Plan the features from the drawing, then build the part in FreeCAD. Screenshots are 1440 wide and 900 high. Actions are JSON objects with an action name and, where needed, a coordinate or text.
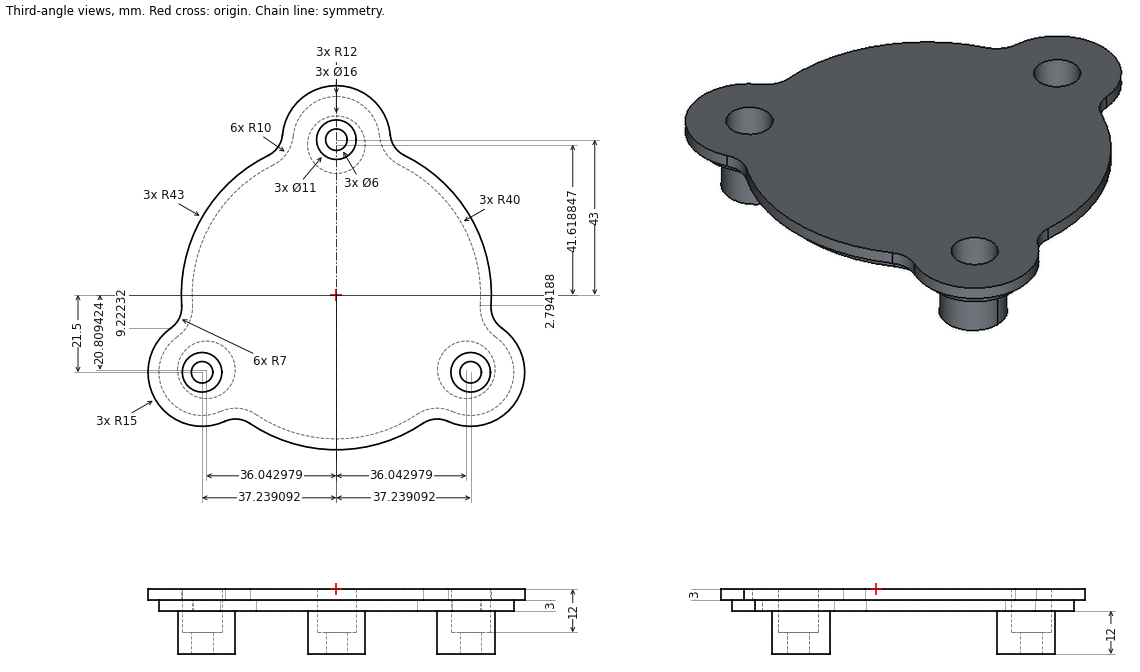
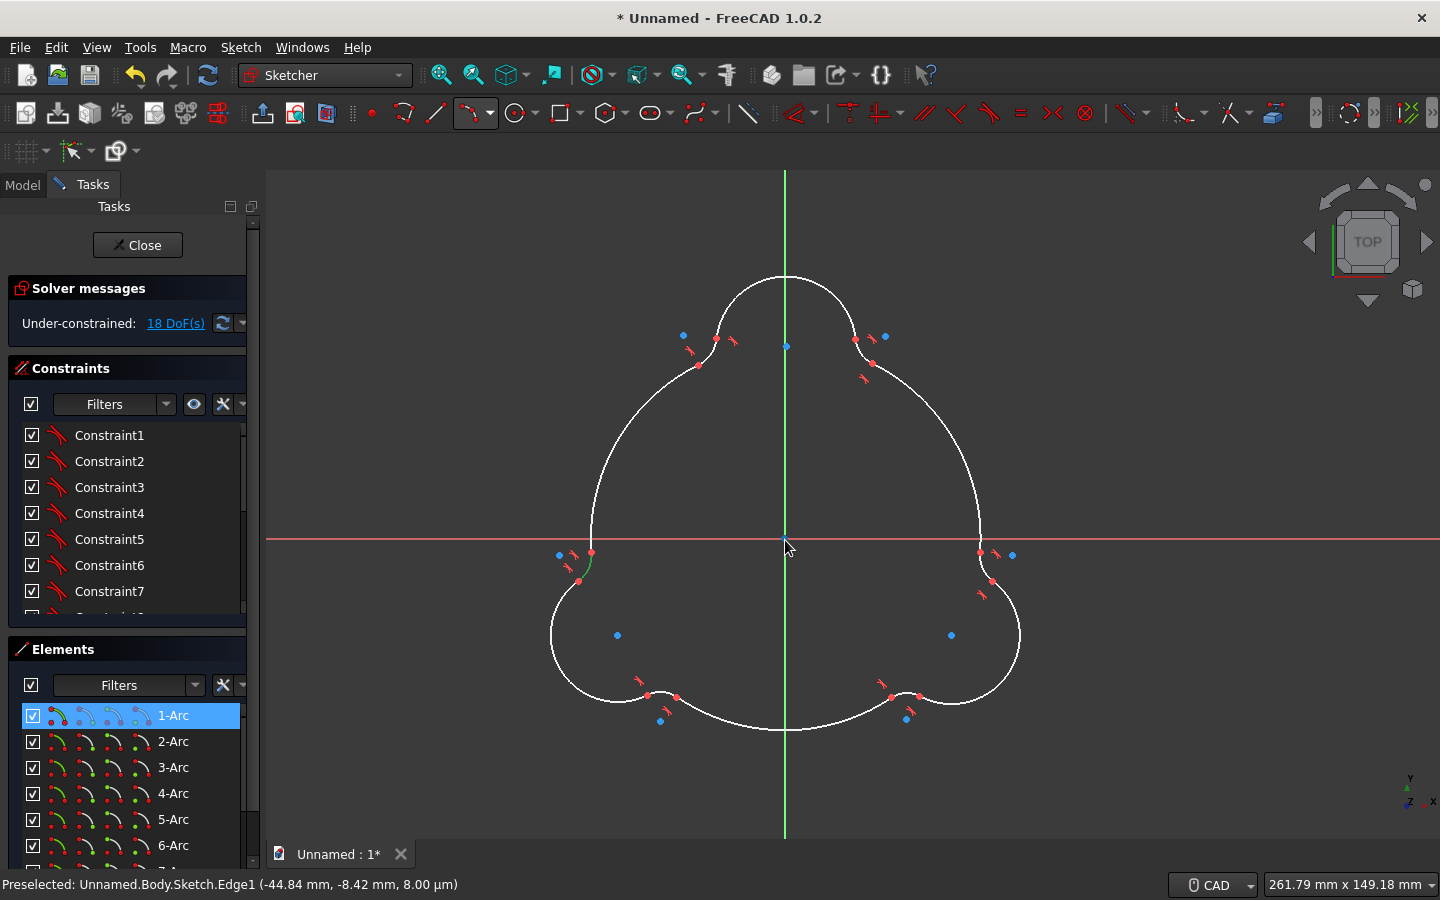
{"action": "scroll", "coordinate": [669, 693], "scroll_direction": "up", "scroll_amount": 2}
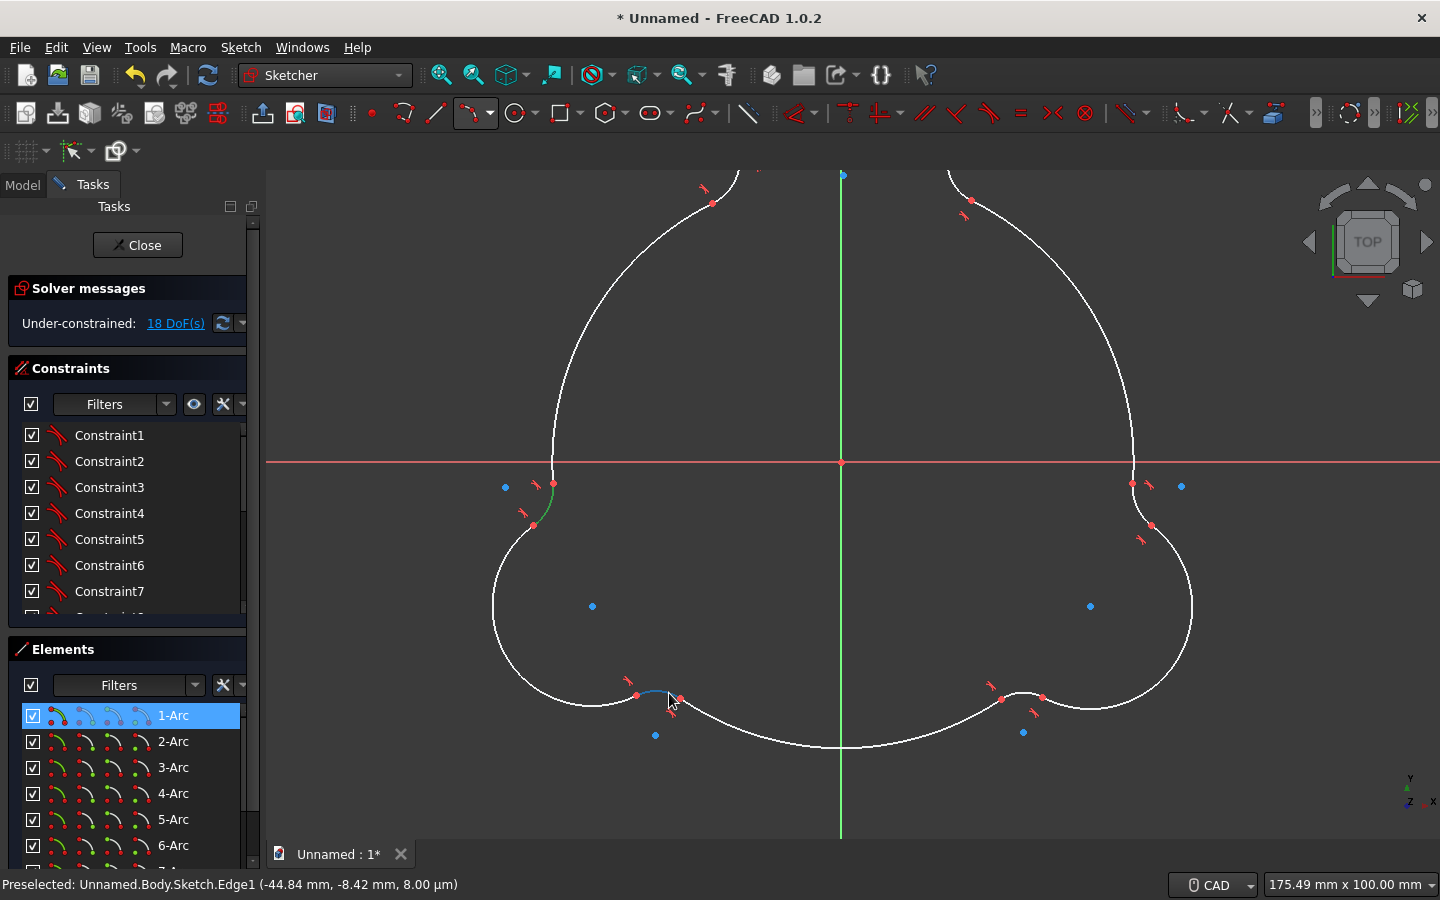
{"action": "left_click", "coordinate": [668, 693]}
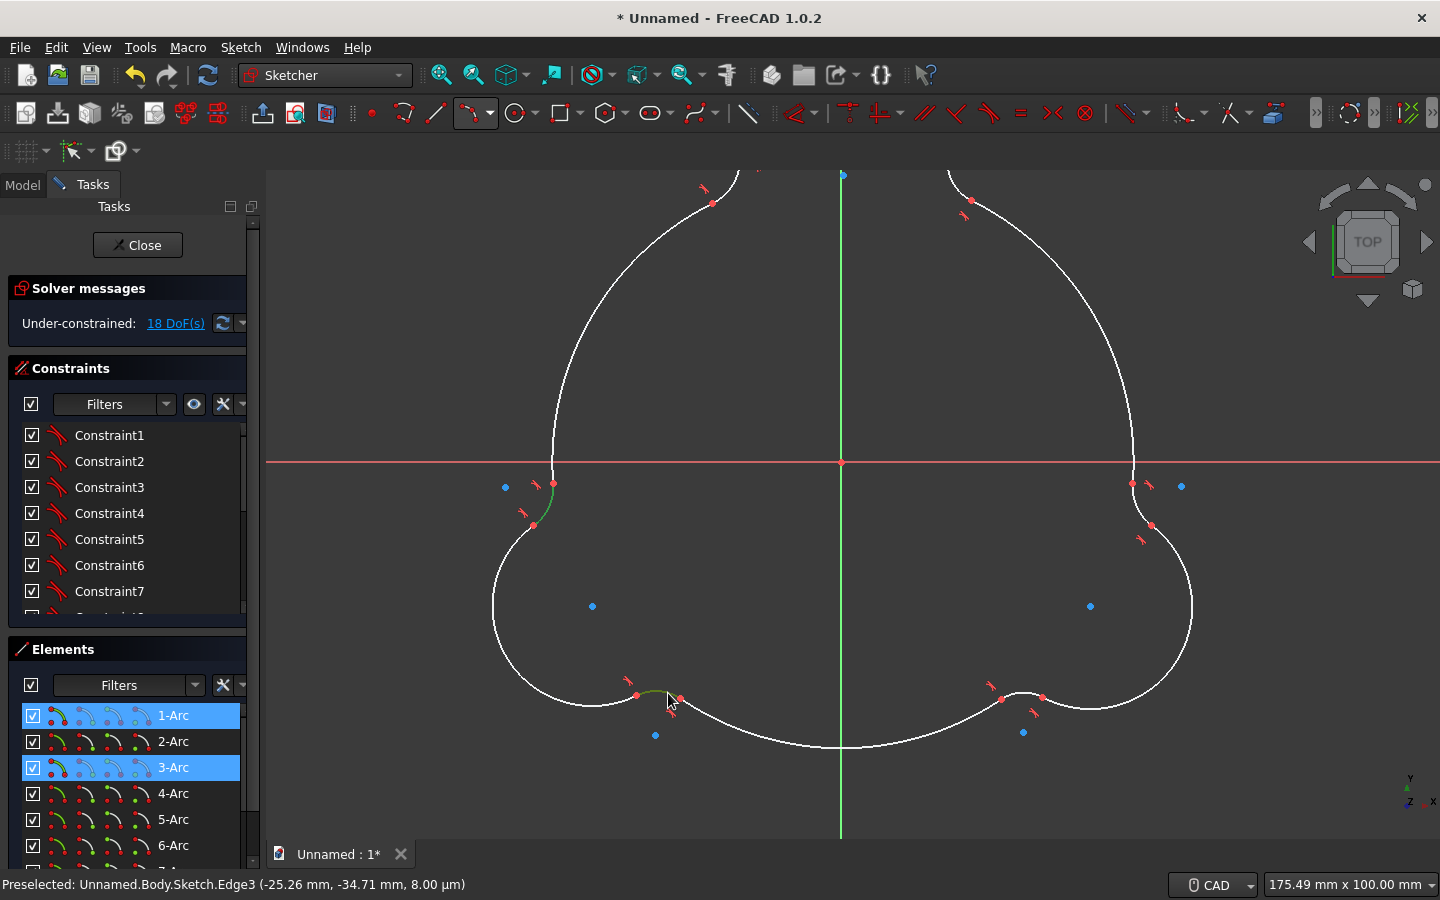
{"action": "left_click", "coordinate": [1030, 693]}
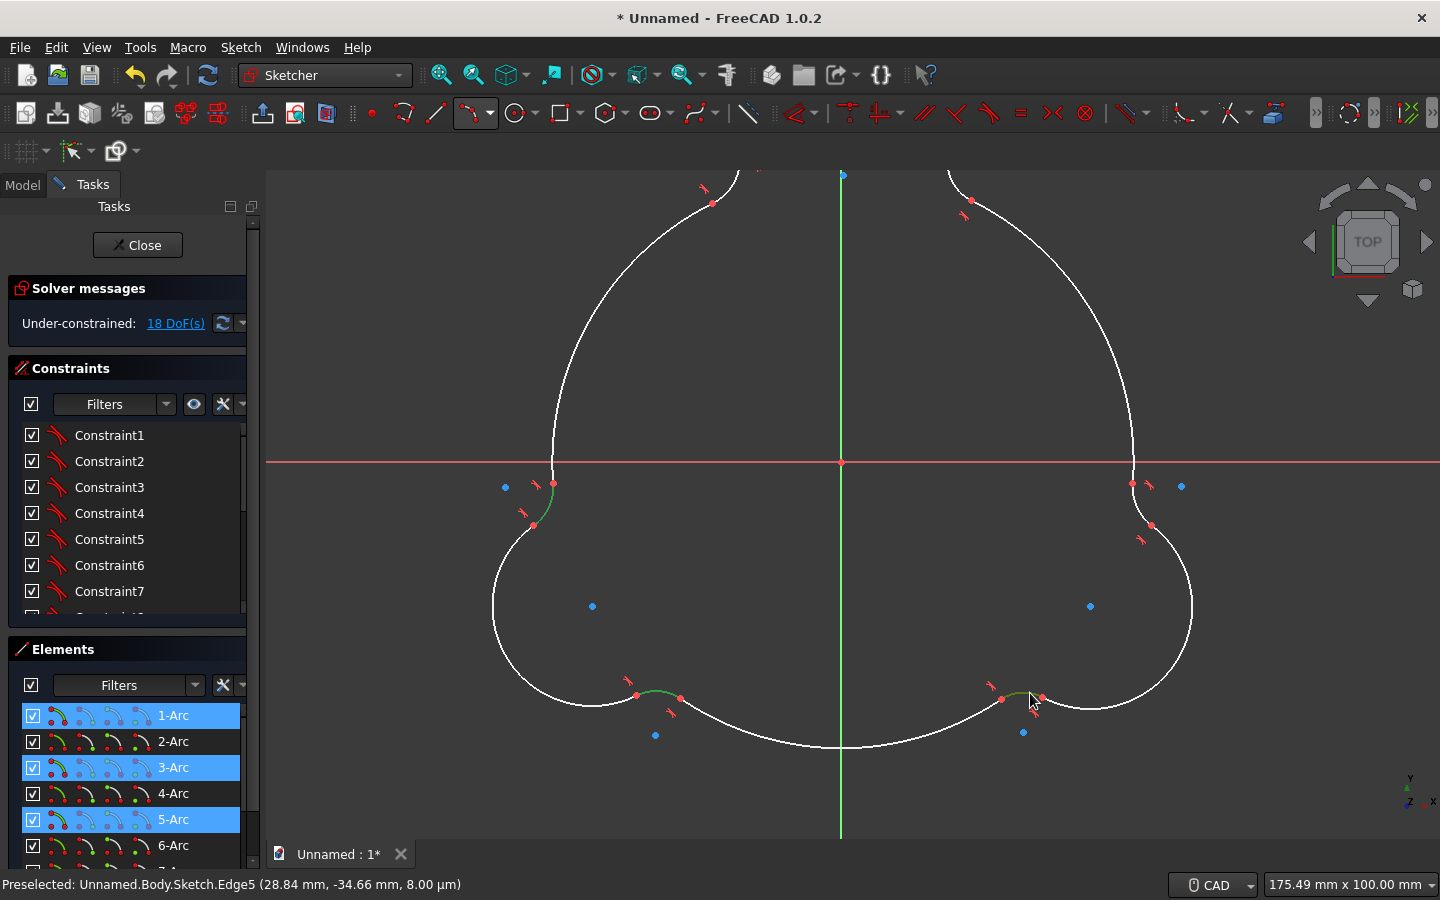
{"action": "left_click", "coordinate": [1134, 498]}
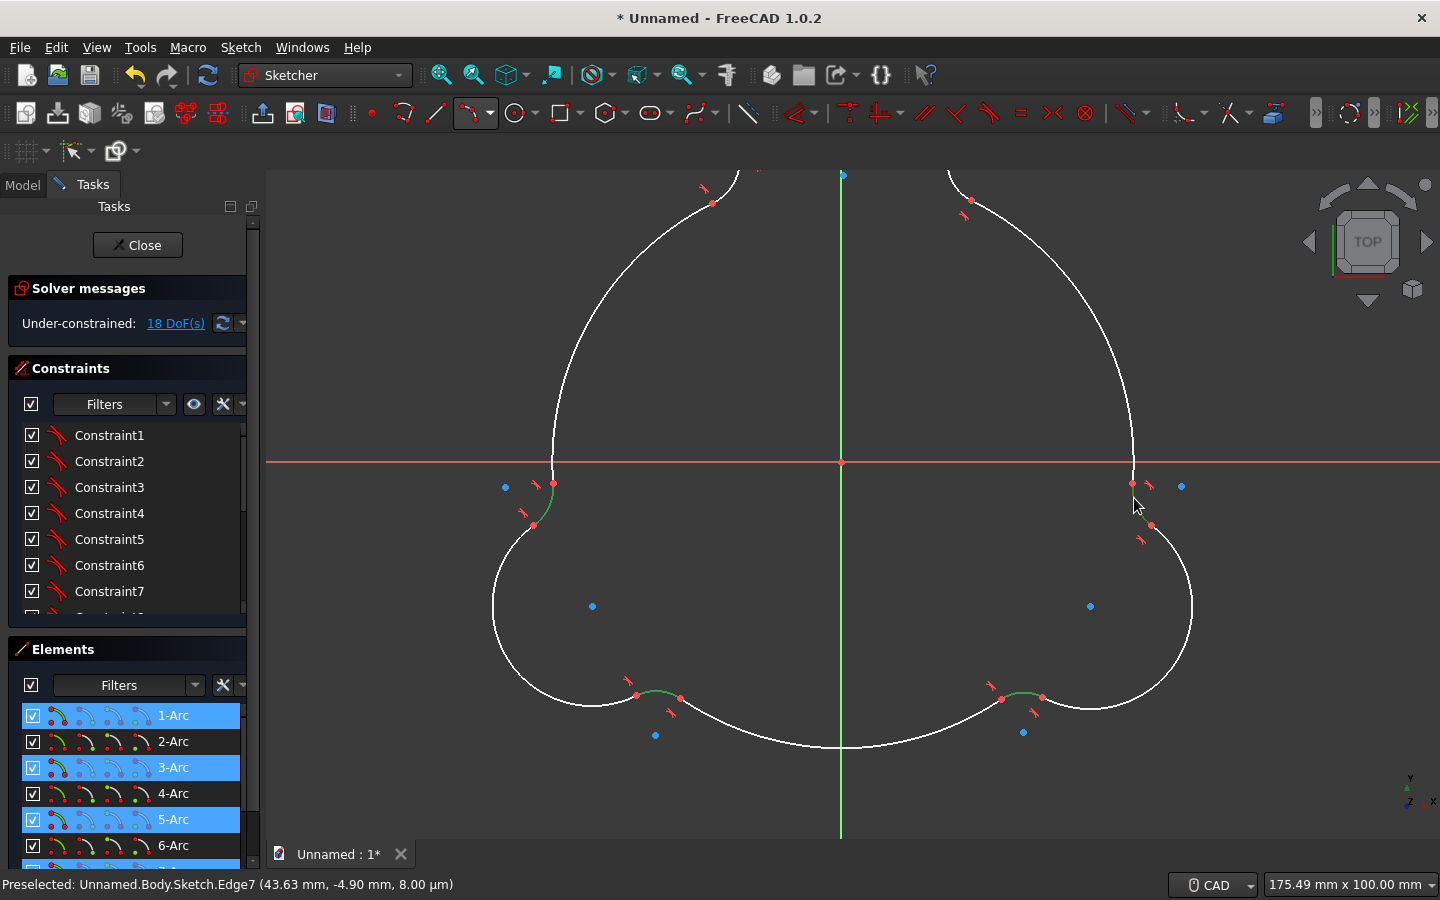
{"action": "scroll", "coordinate": [669, 693], "scroll_direction": "down", "scroll_amount": 2}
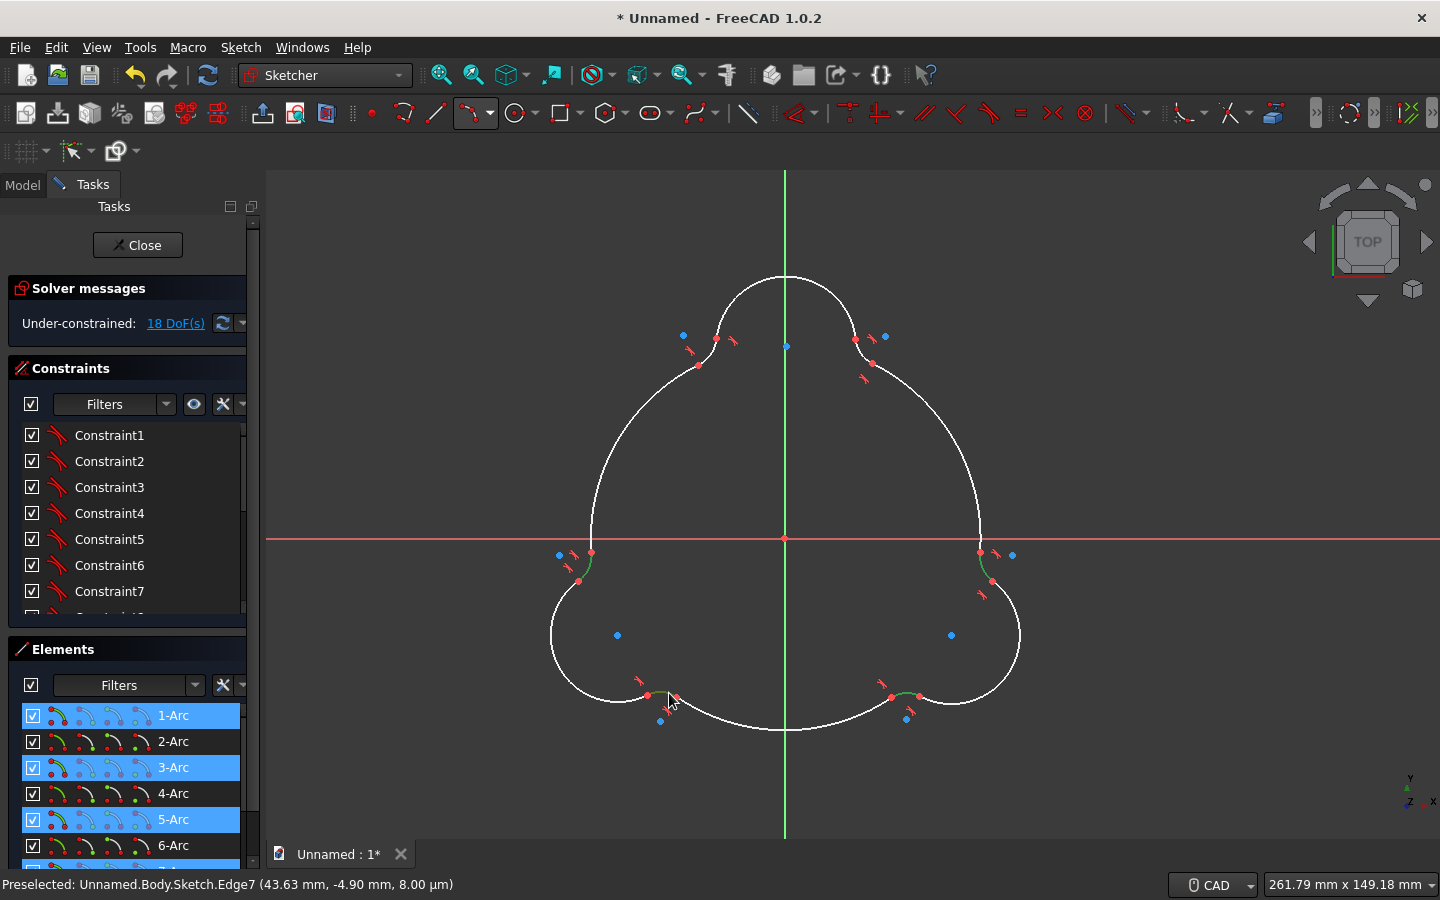
{"action": "scroll", "coordinate": [858, 348], "scroll_direction": "up", "scroll_amount": 3}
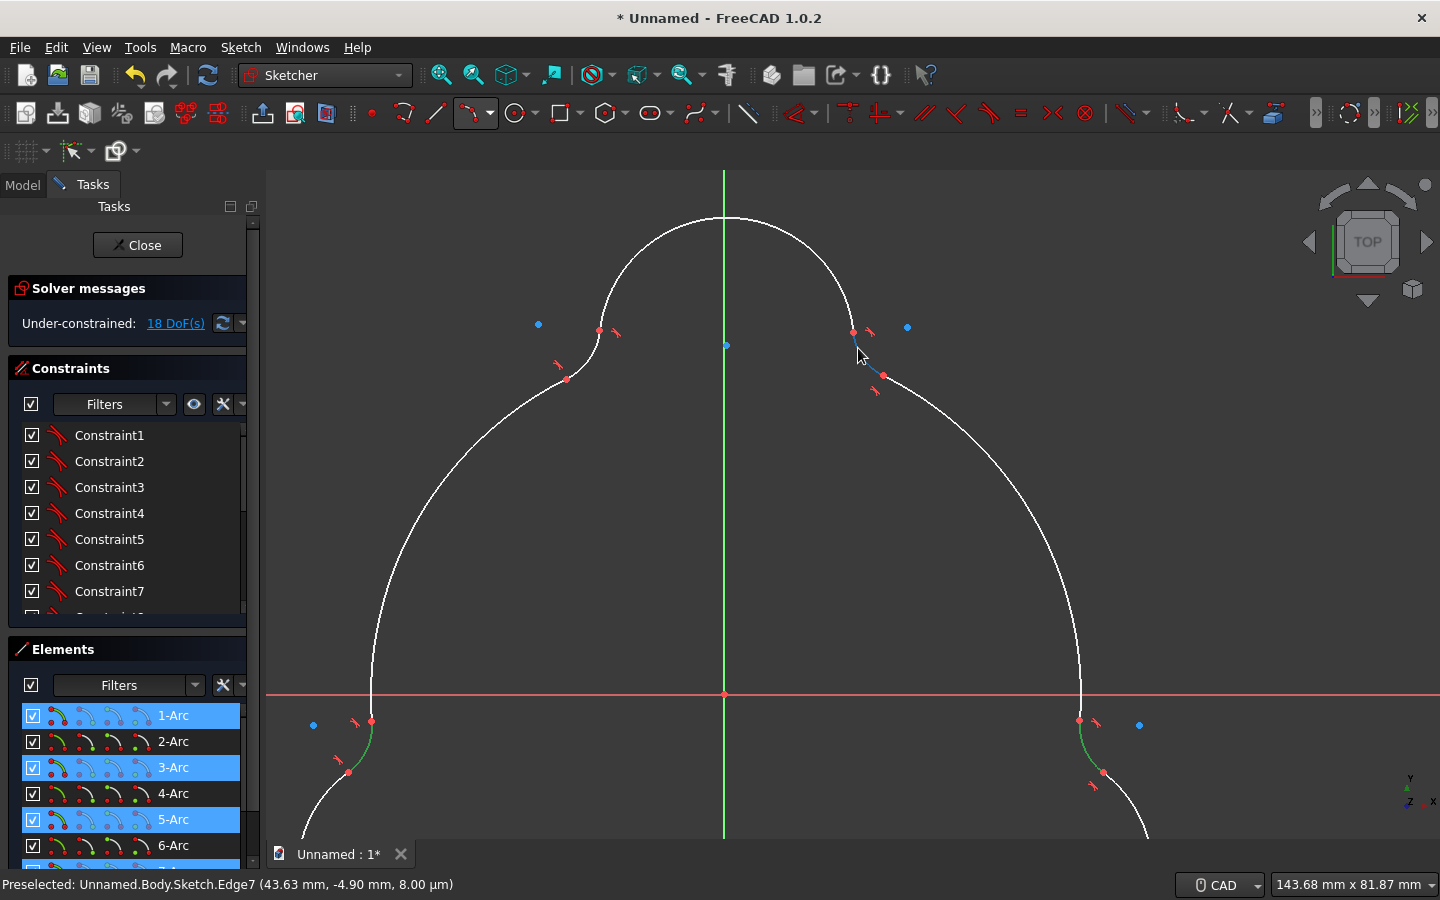
{"action": "left_click", "coordinate": [858, 348]}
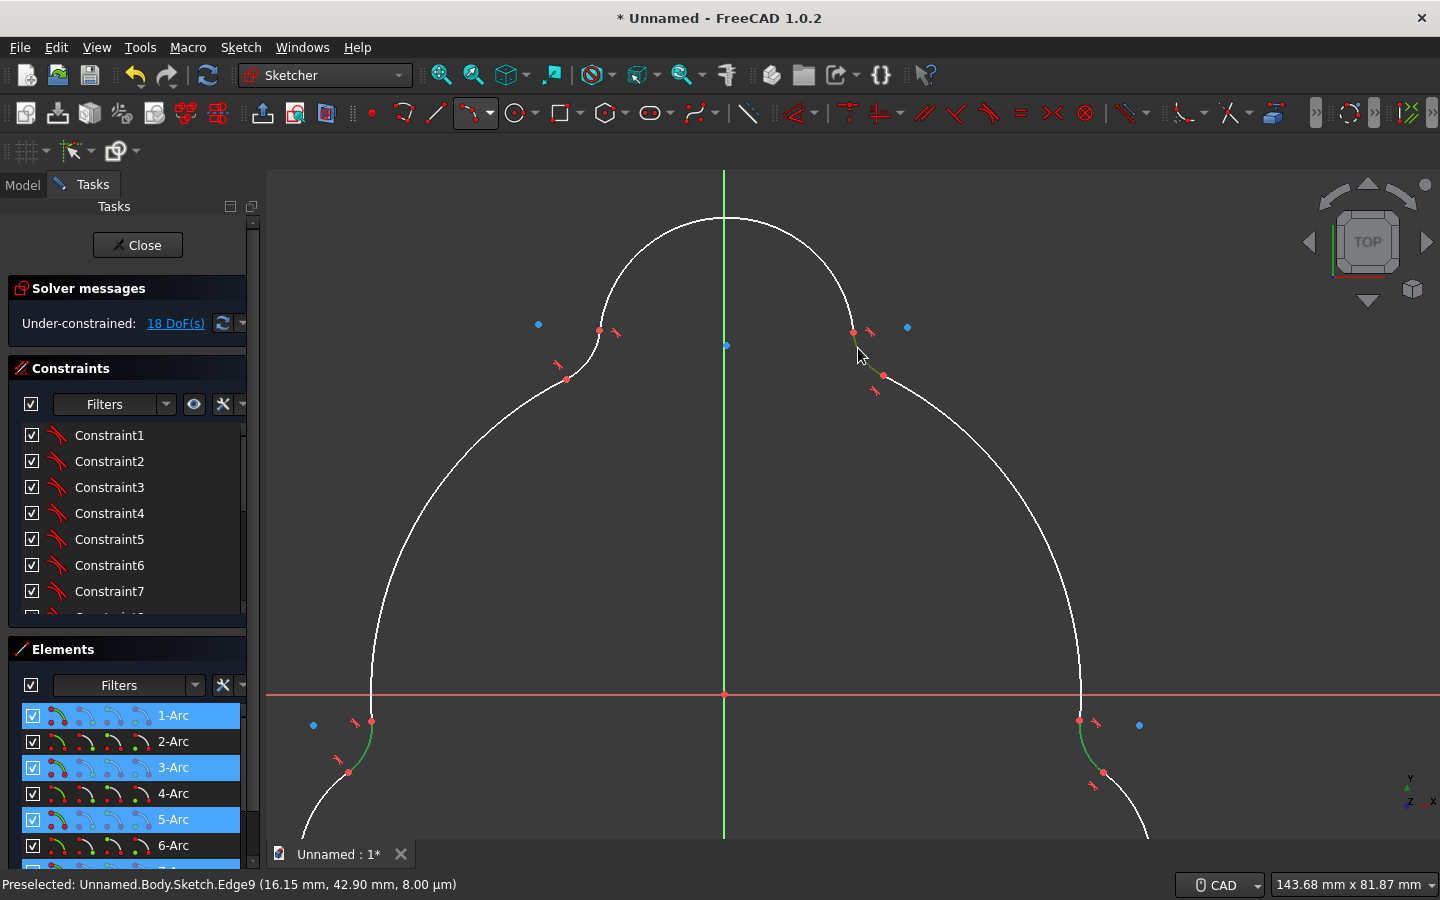
{"action": "left_click", "coordinate": [581, 369]}